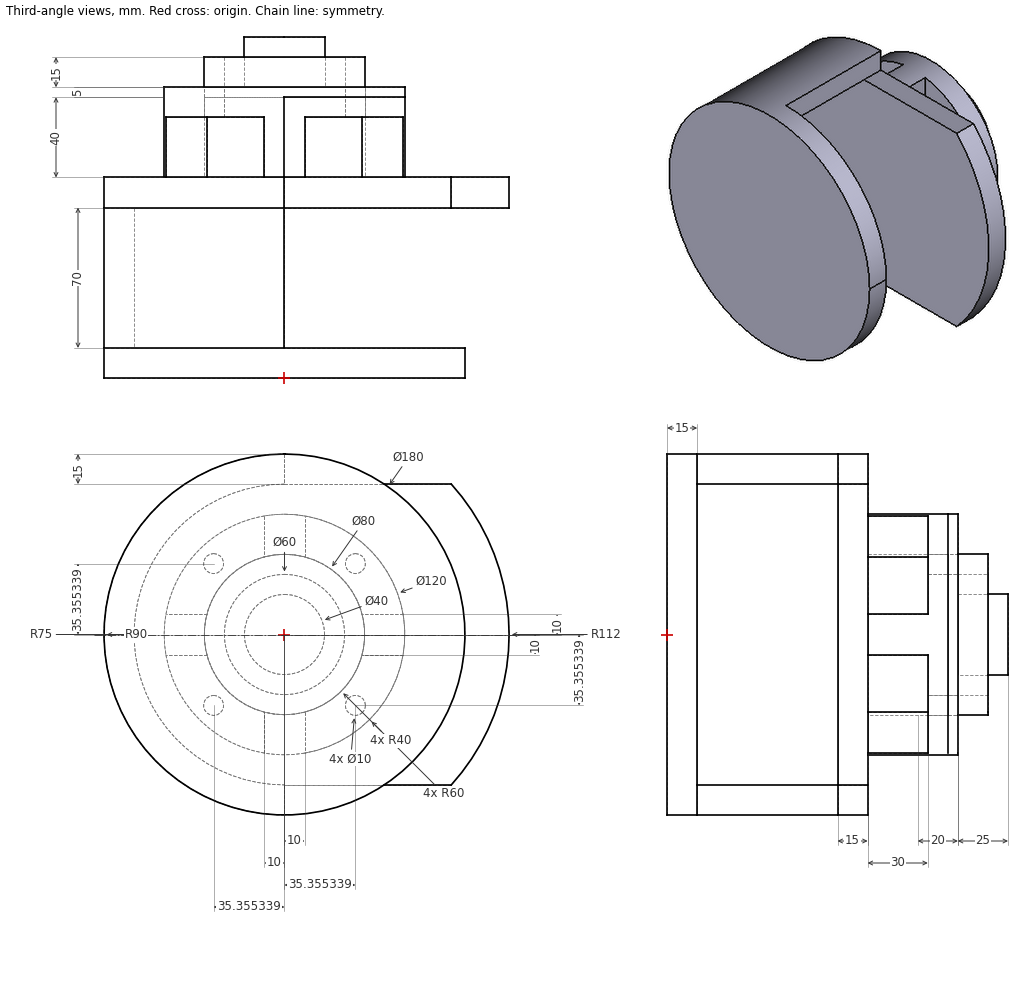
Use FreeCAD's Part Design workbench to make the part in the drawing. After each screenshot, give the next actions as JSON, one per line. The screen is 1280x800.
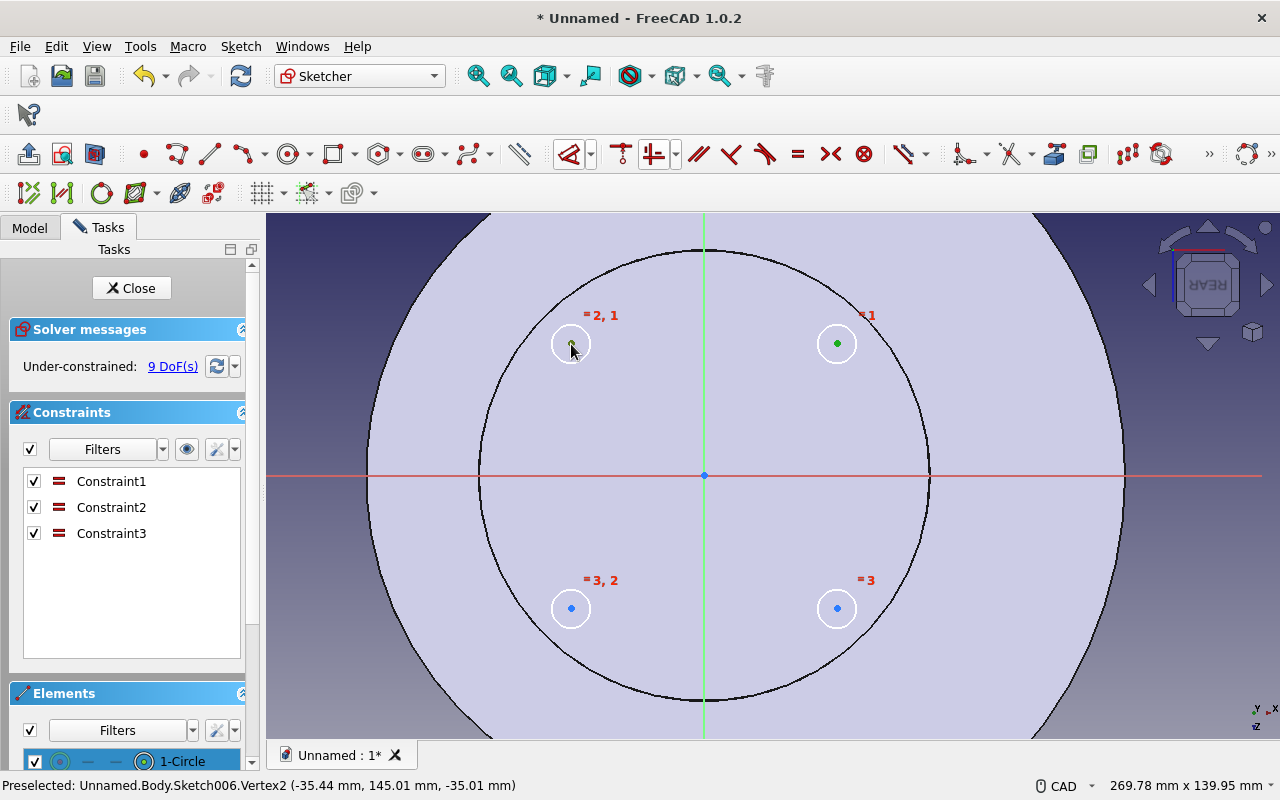
{"action": "key", "text": "h"}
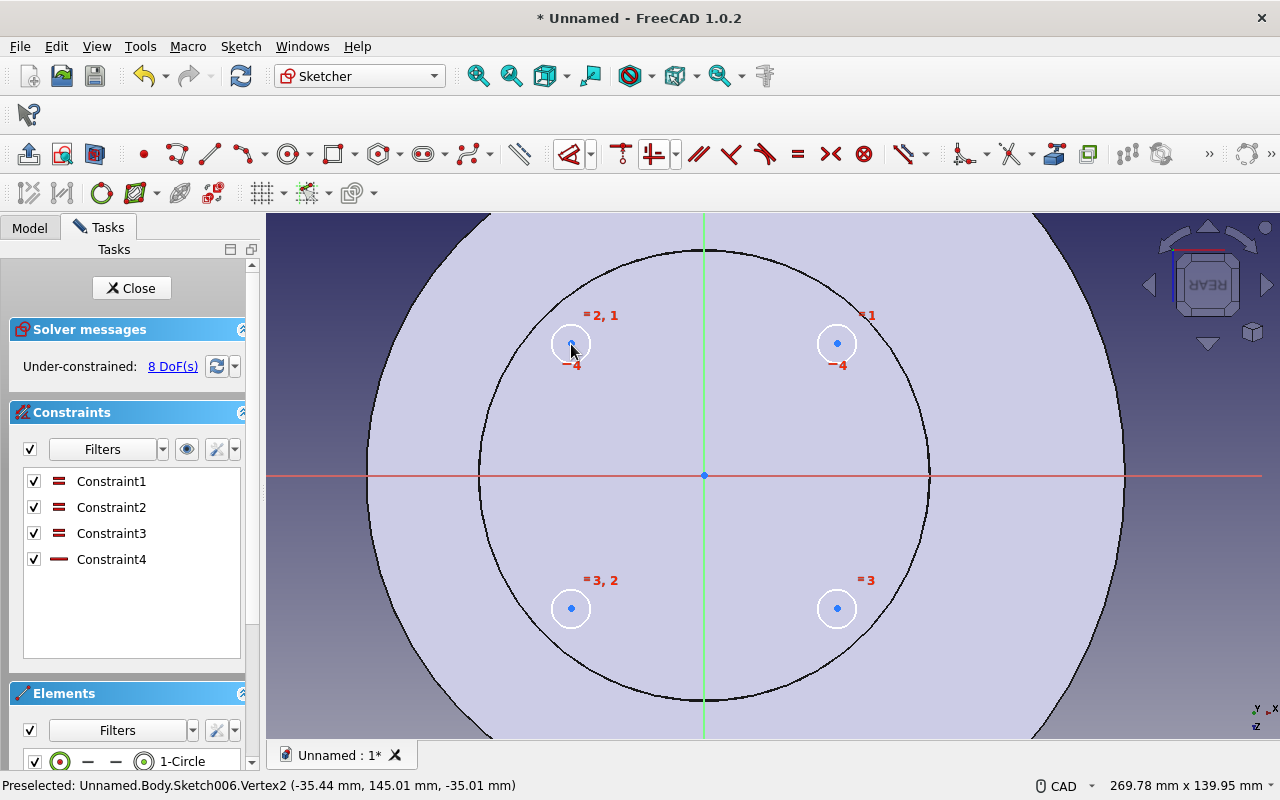
{"action": "left_click", "coordinate": [571, 344]}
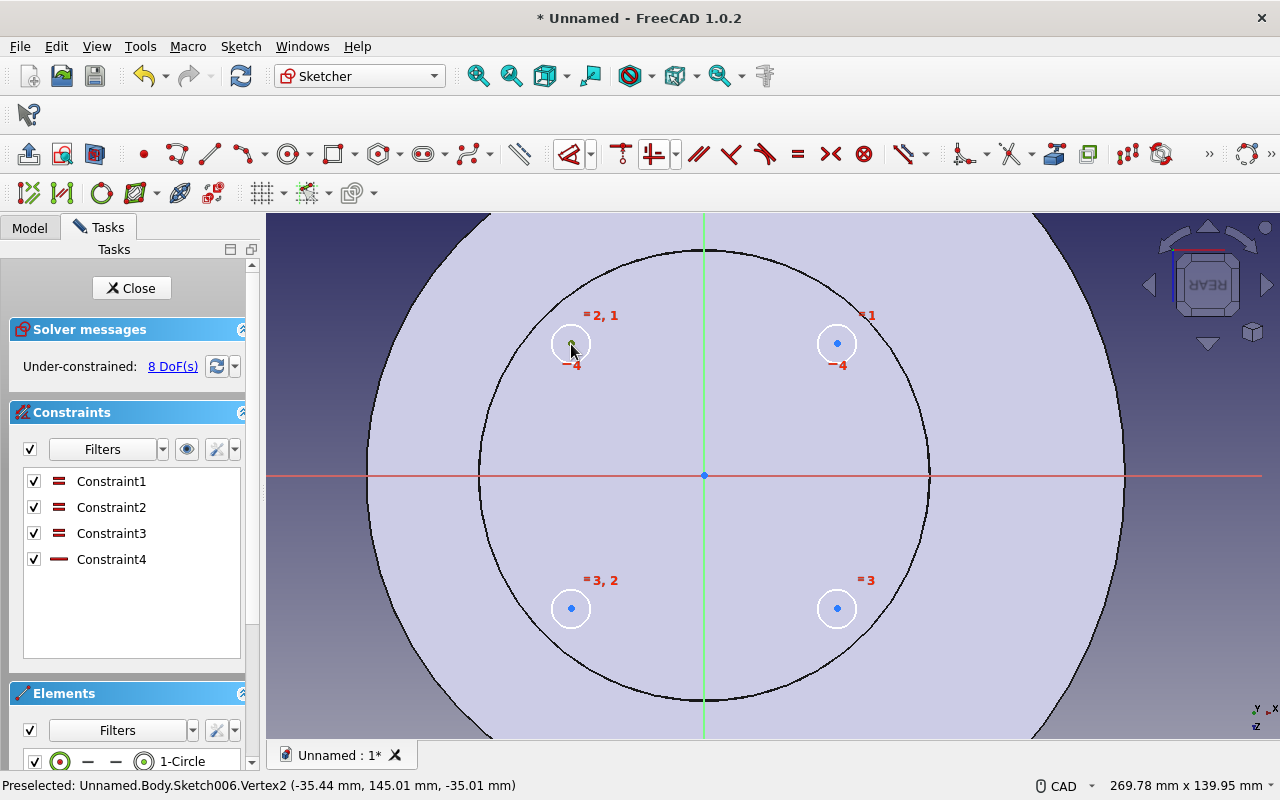
{"action": "left_click", "coordinate": [571, 609]}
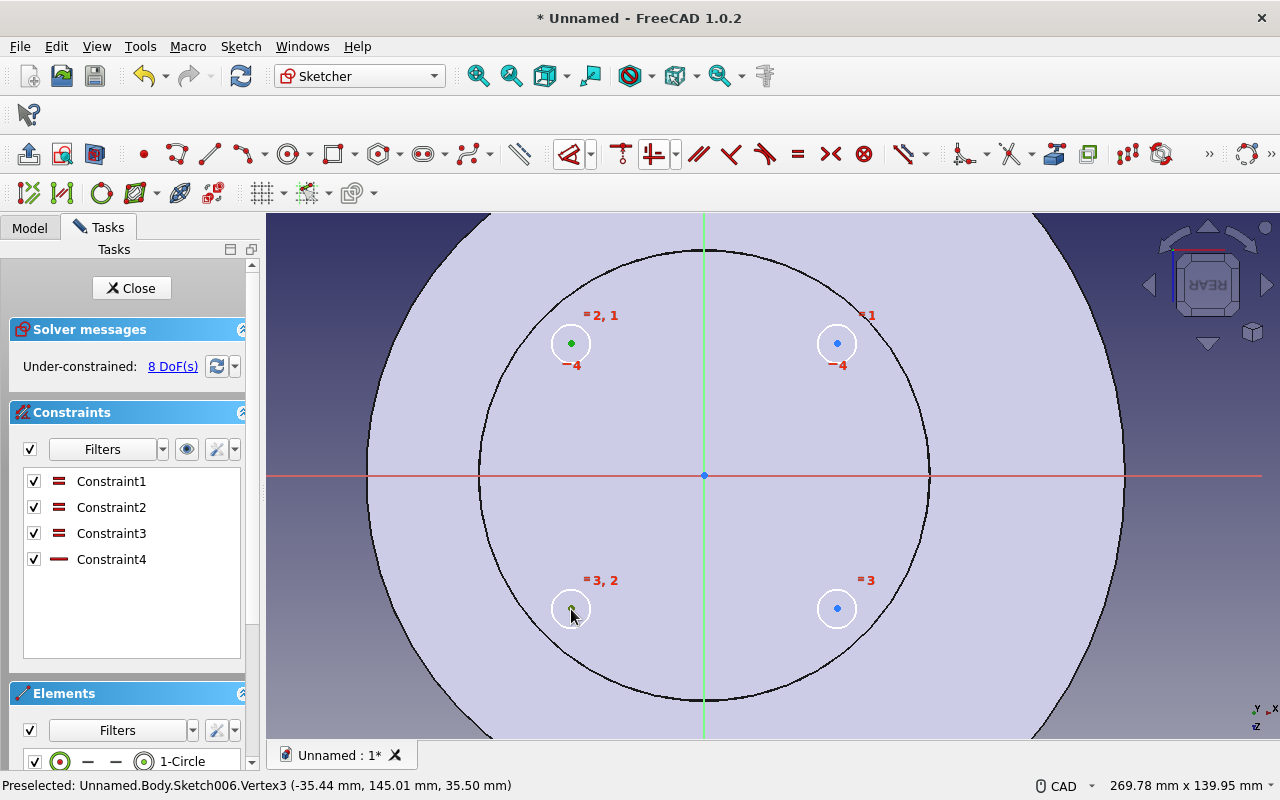
{"action": "left_click", "coordinate": [676, 154]}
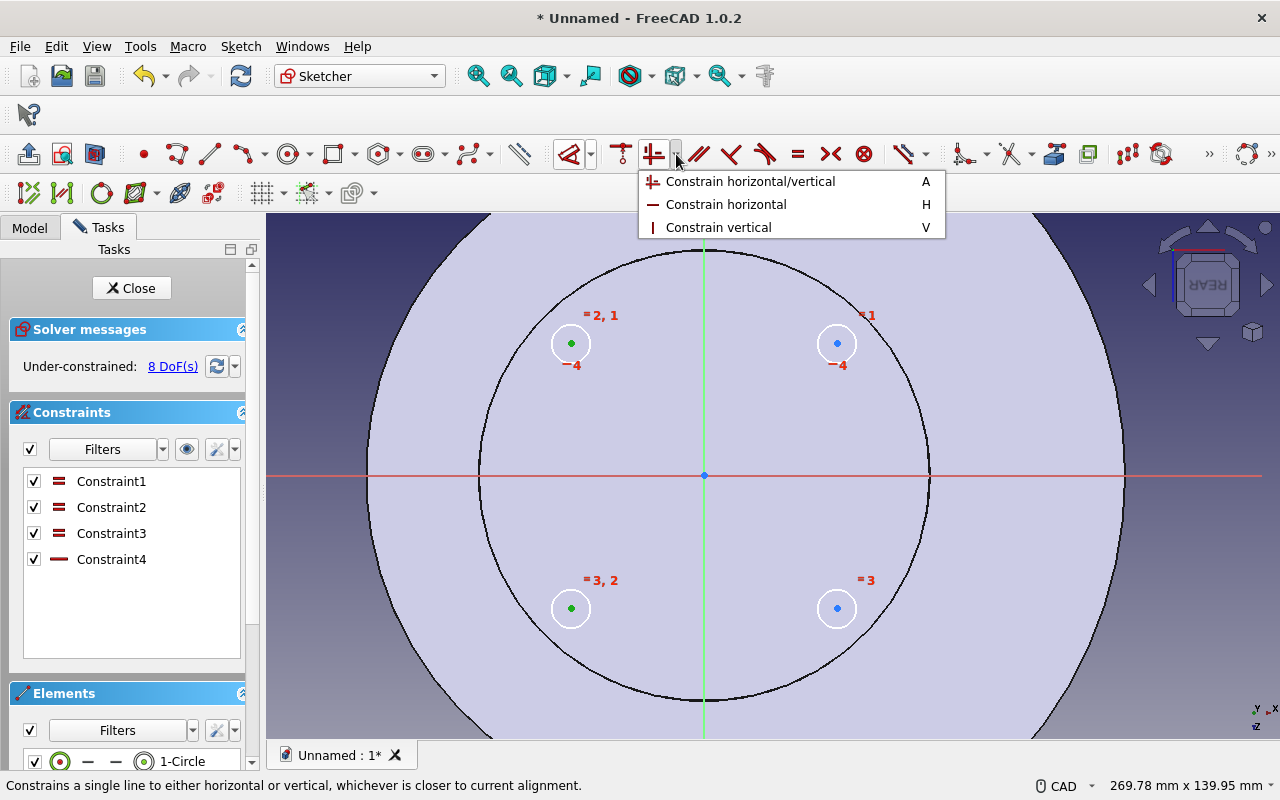
{"action": "left_click", "coordinate": [792, 228]}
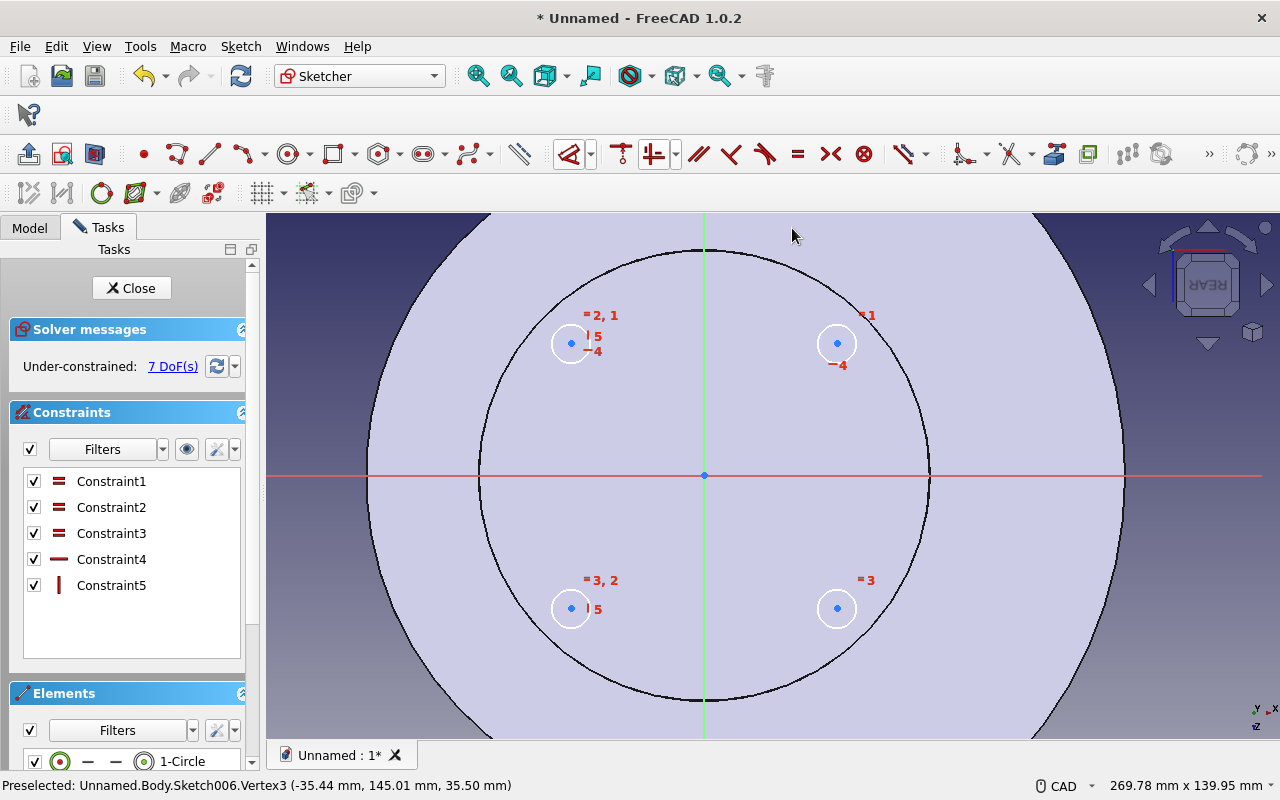
{"action": "left_click", "coordinate": [837, 344]}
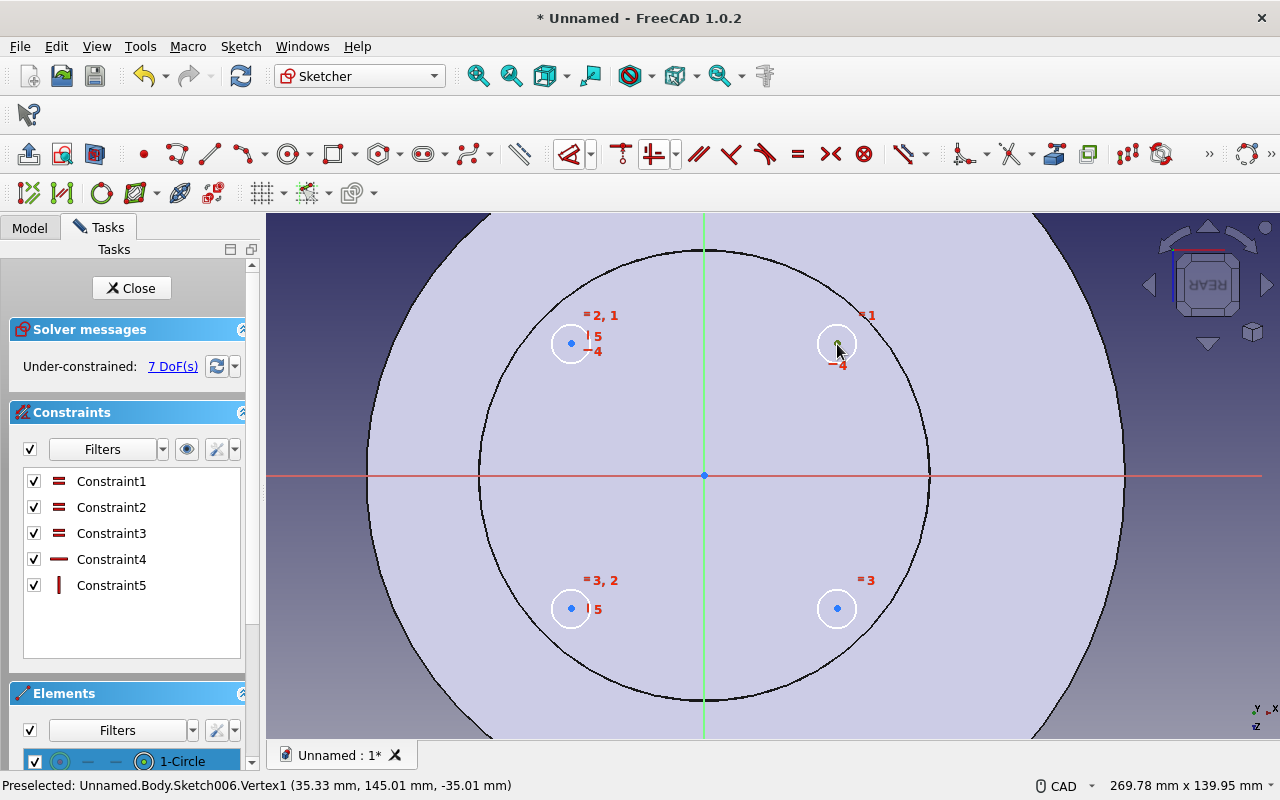
{"action": "left_click", "coordinate": [837, 609]}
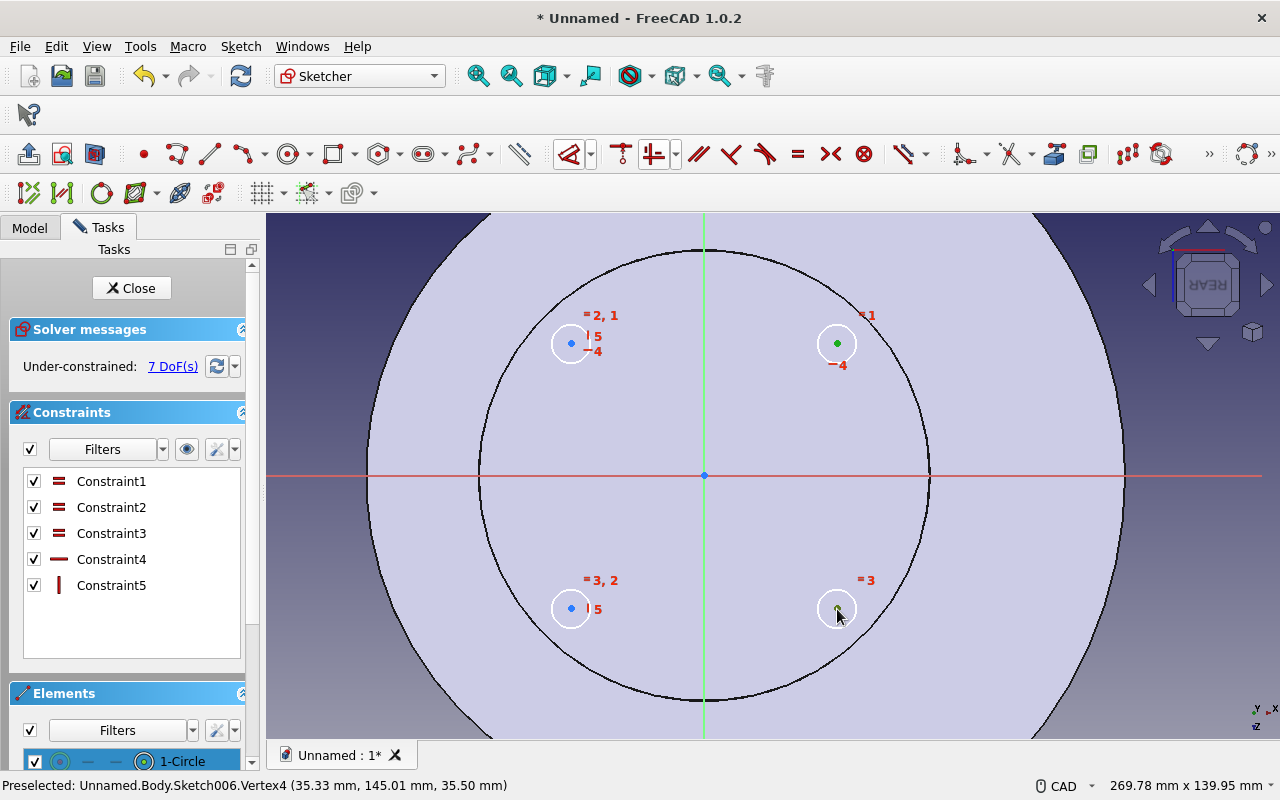
{"action": "left_click", "coordinate": [676, 154]}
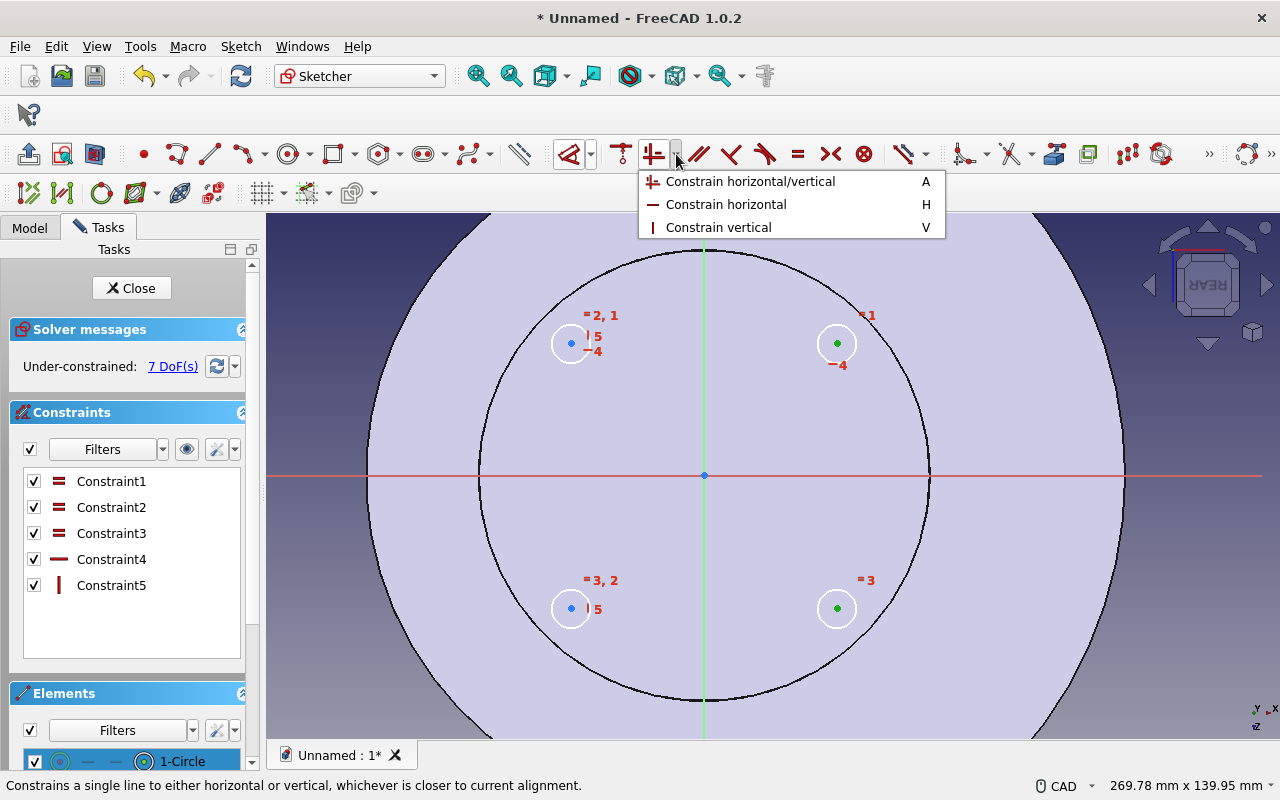
{"action": "left_click", "coordinate": [792, 228]}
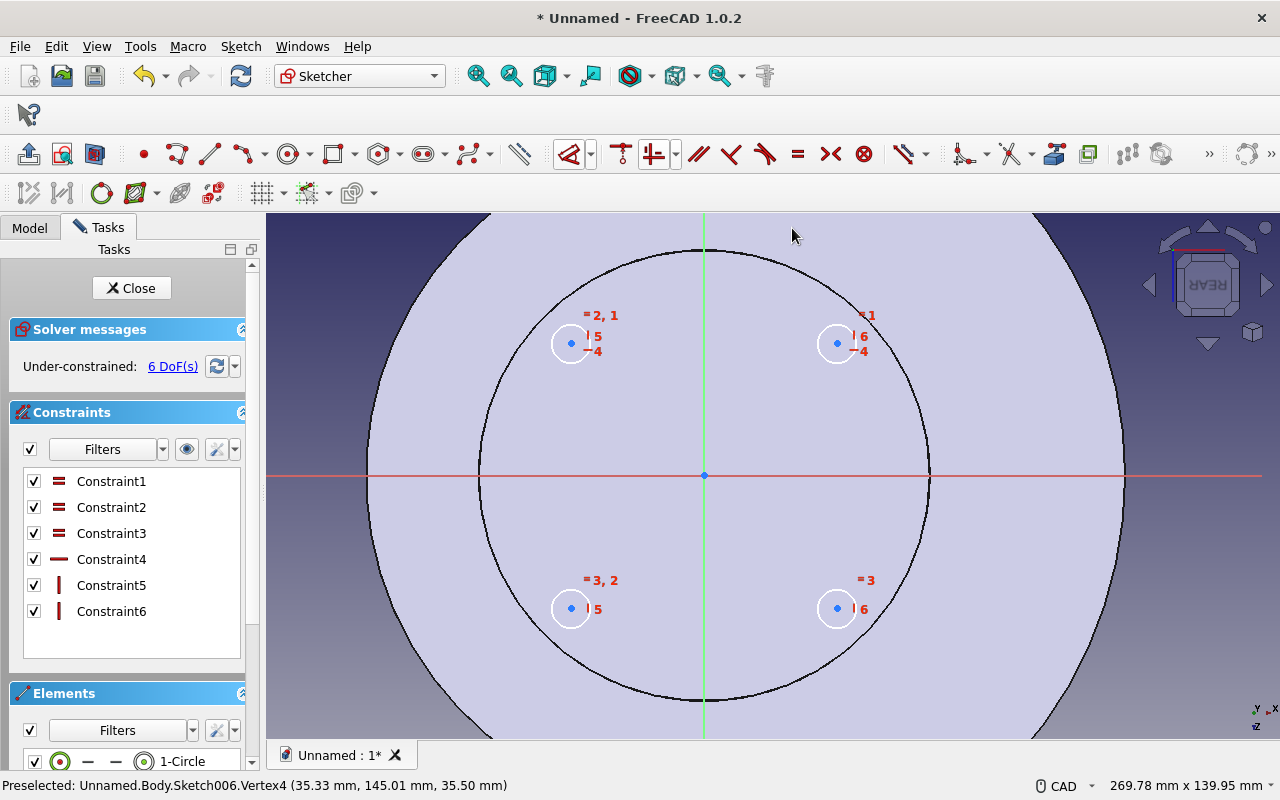
{"action": "left_click", "coordinate": [571, 609]}